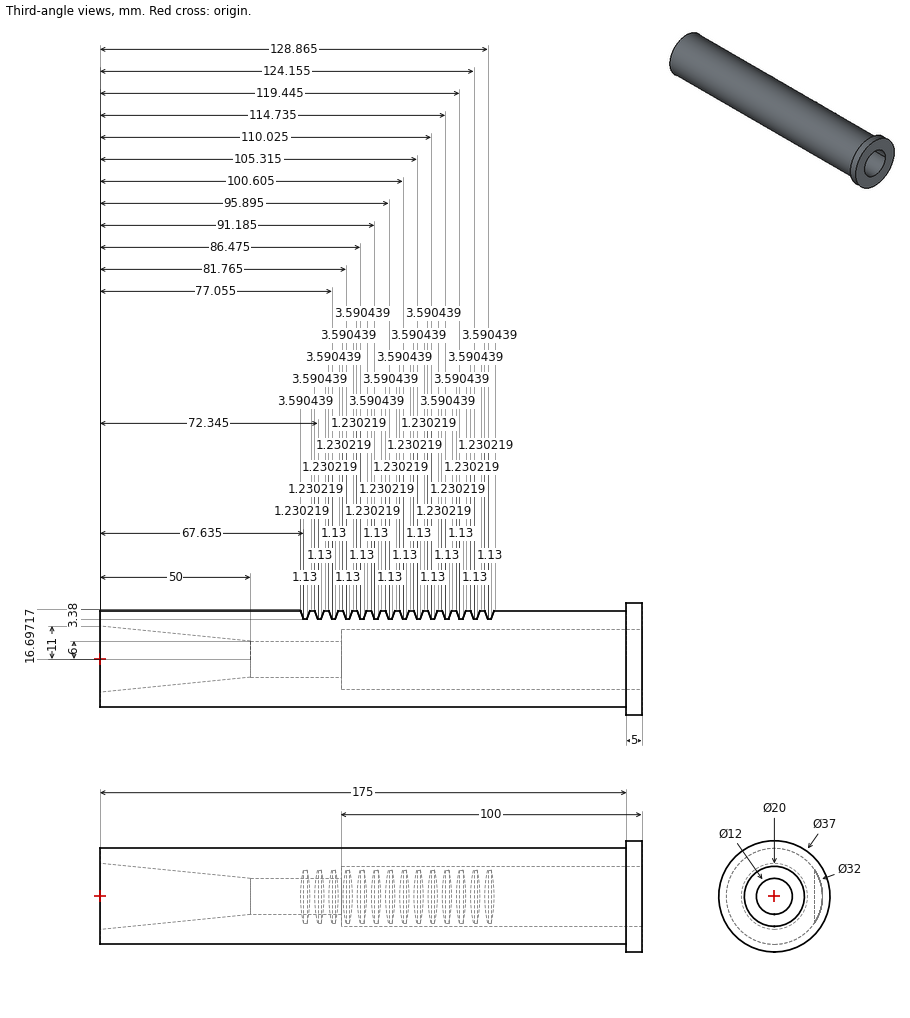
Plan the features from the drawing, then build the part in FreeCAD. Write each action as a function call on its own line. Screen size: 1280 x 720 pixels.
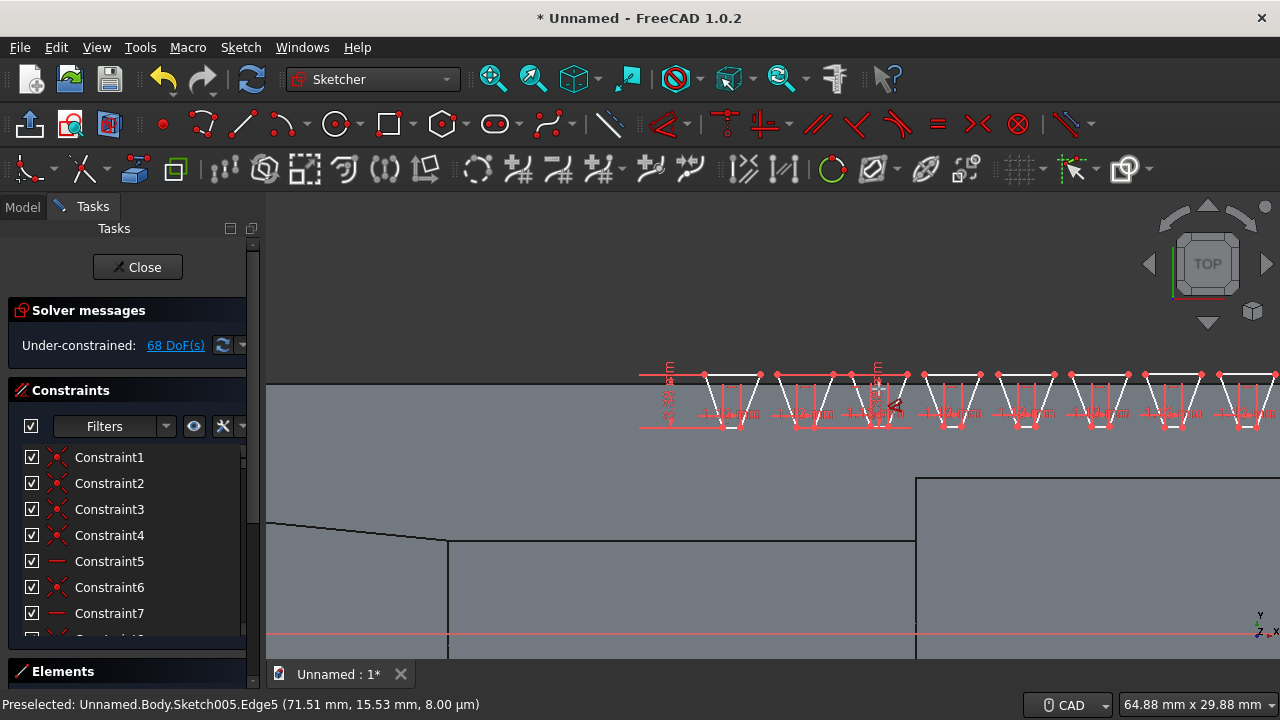
click(857, 391)
click(953, 389)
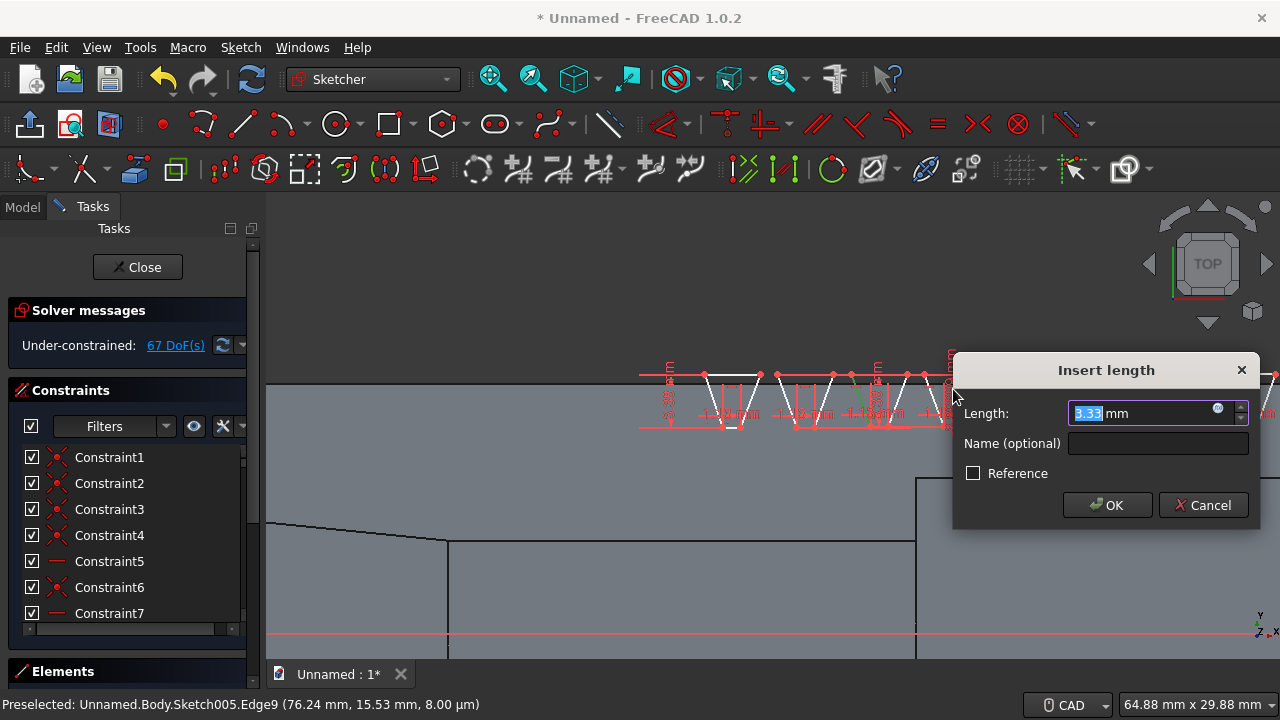
text(3.38)
key(Return)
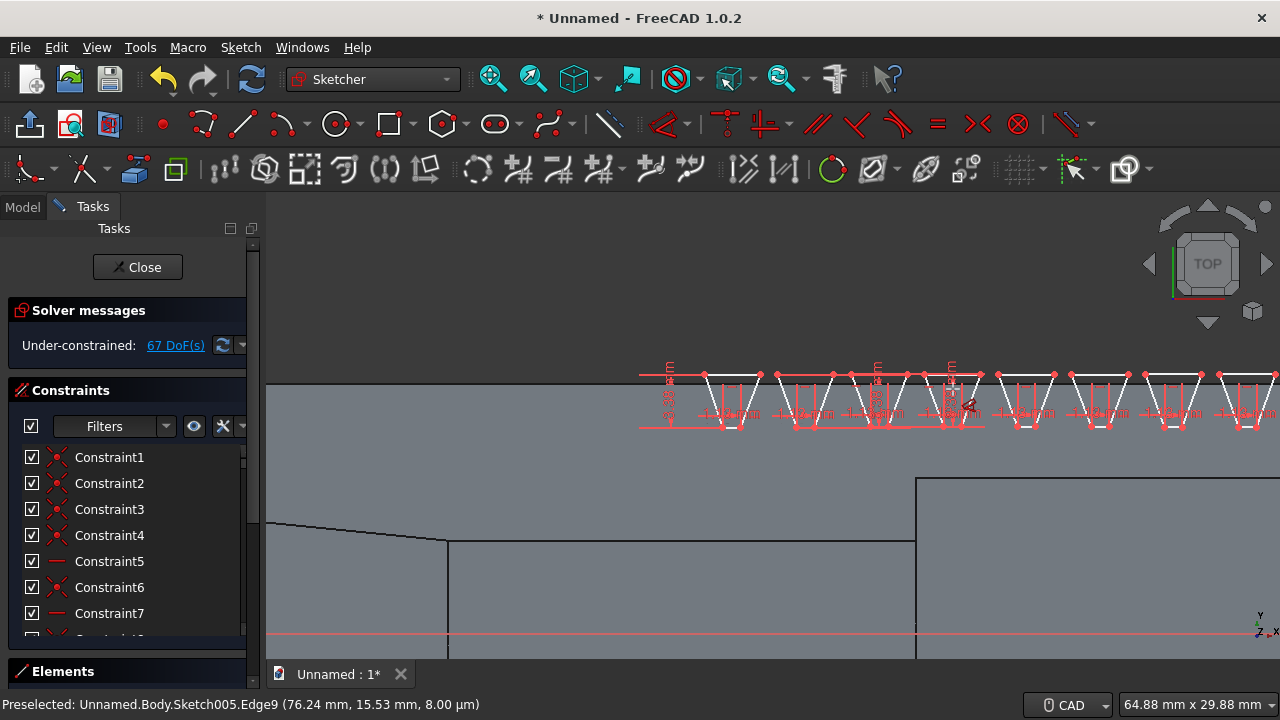
click(930, 391)
click(1026, 389)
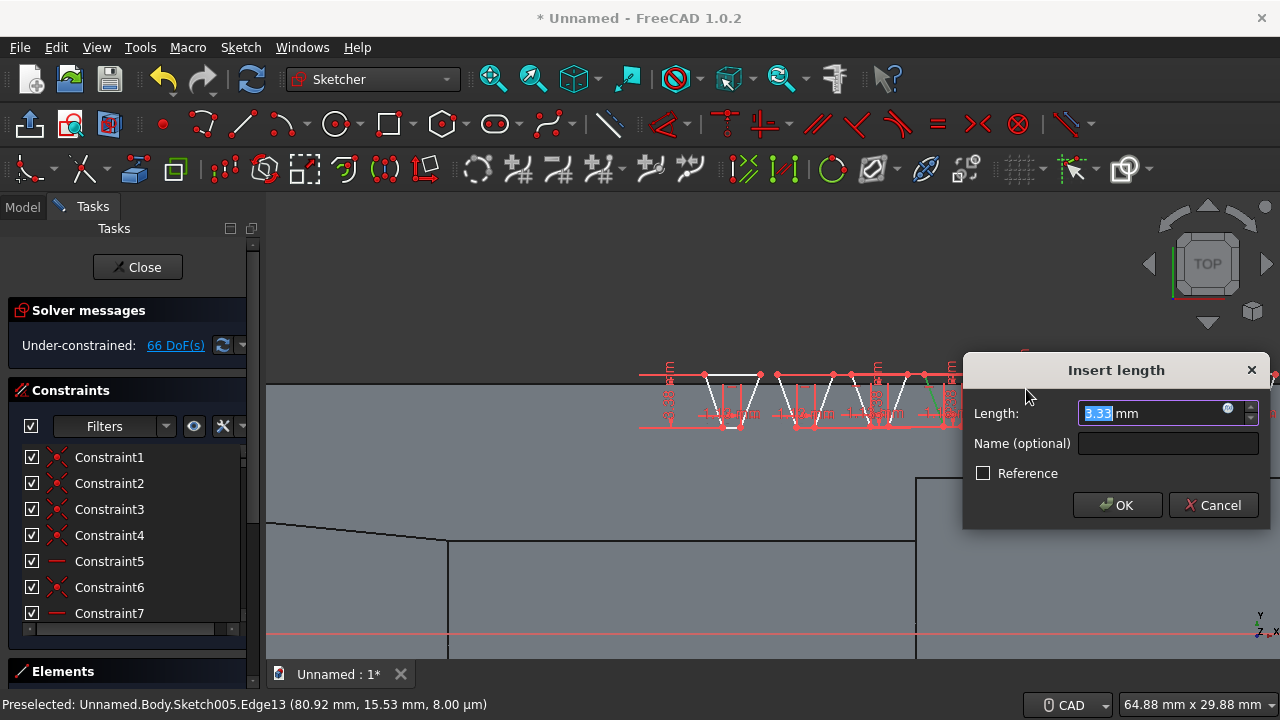
text(3.38)
key(Return)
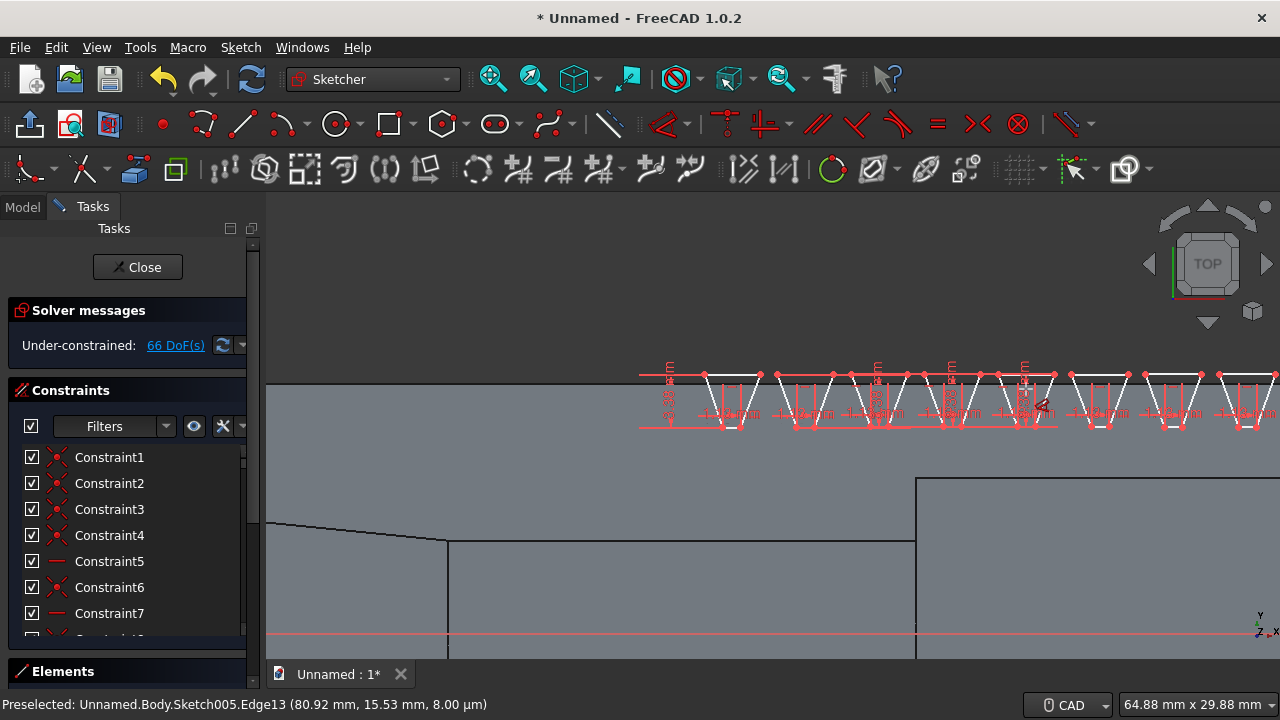
click(1004, 391)
click(1100, 389)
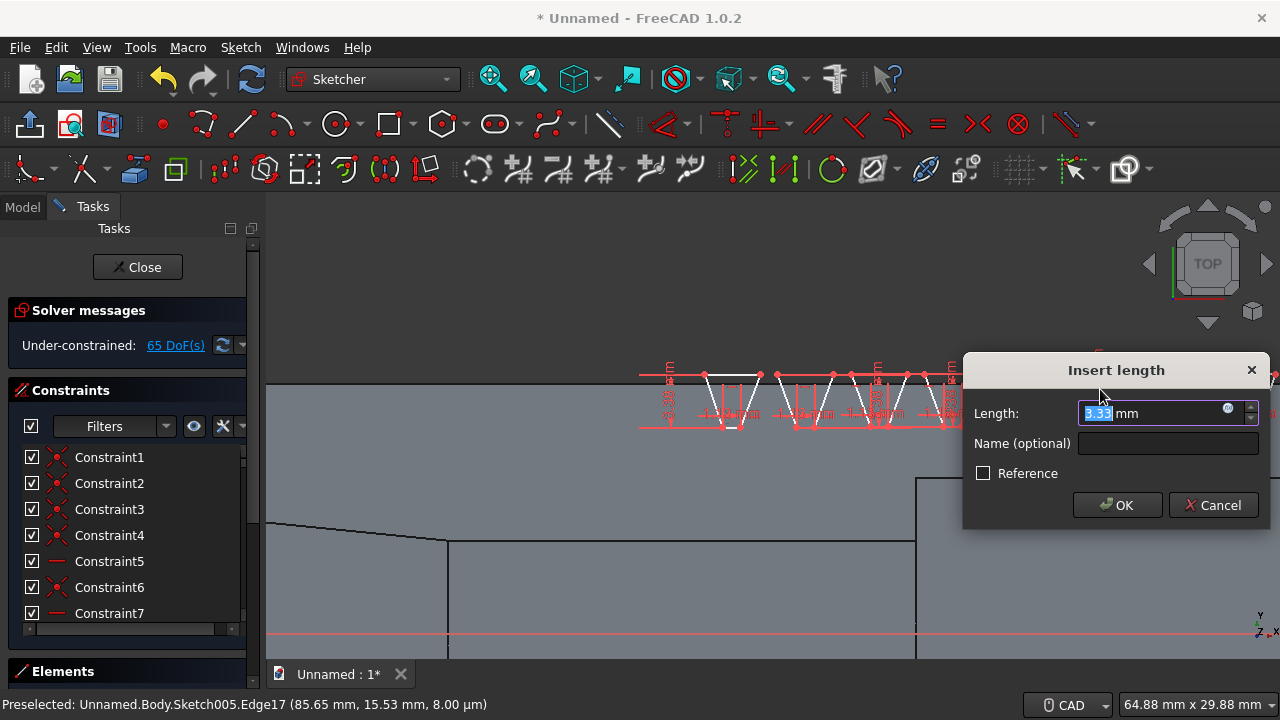
text(3.38)
key(Return)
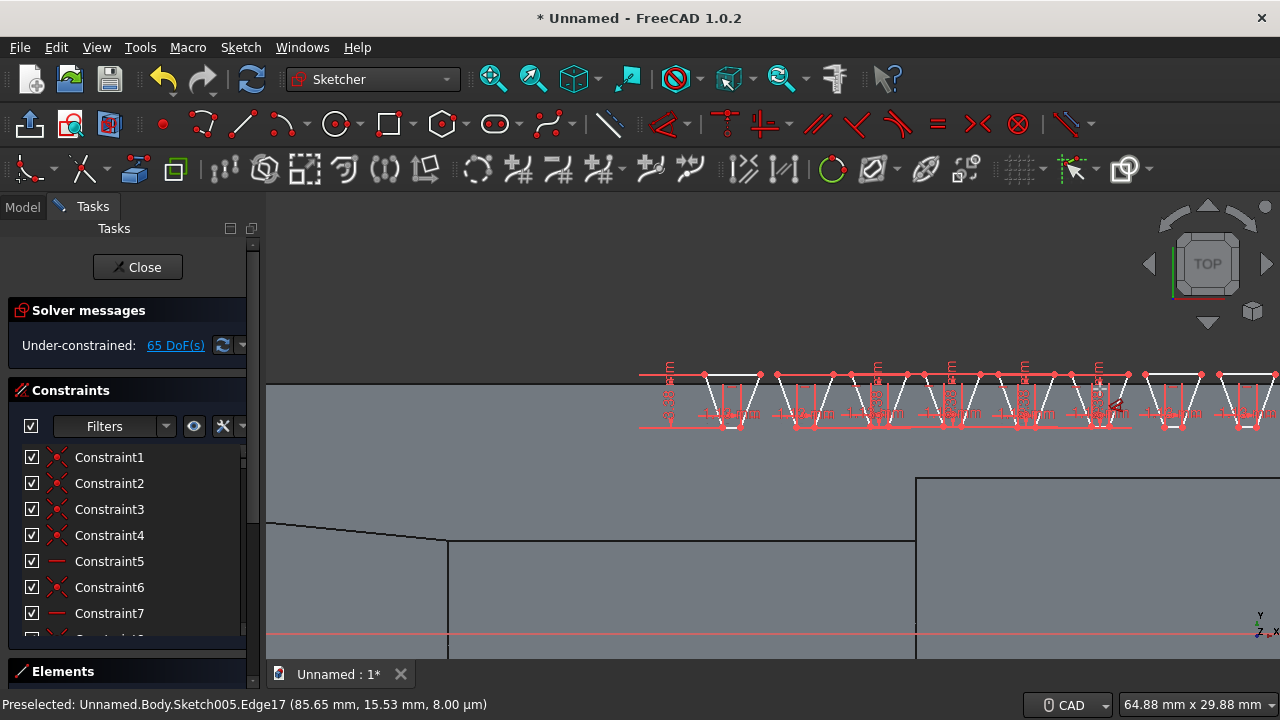
click(1078, 391)
click(1038, 401)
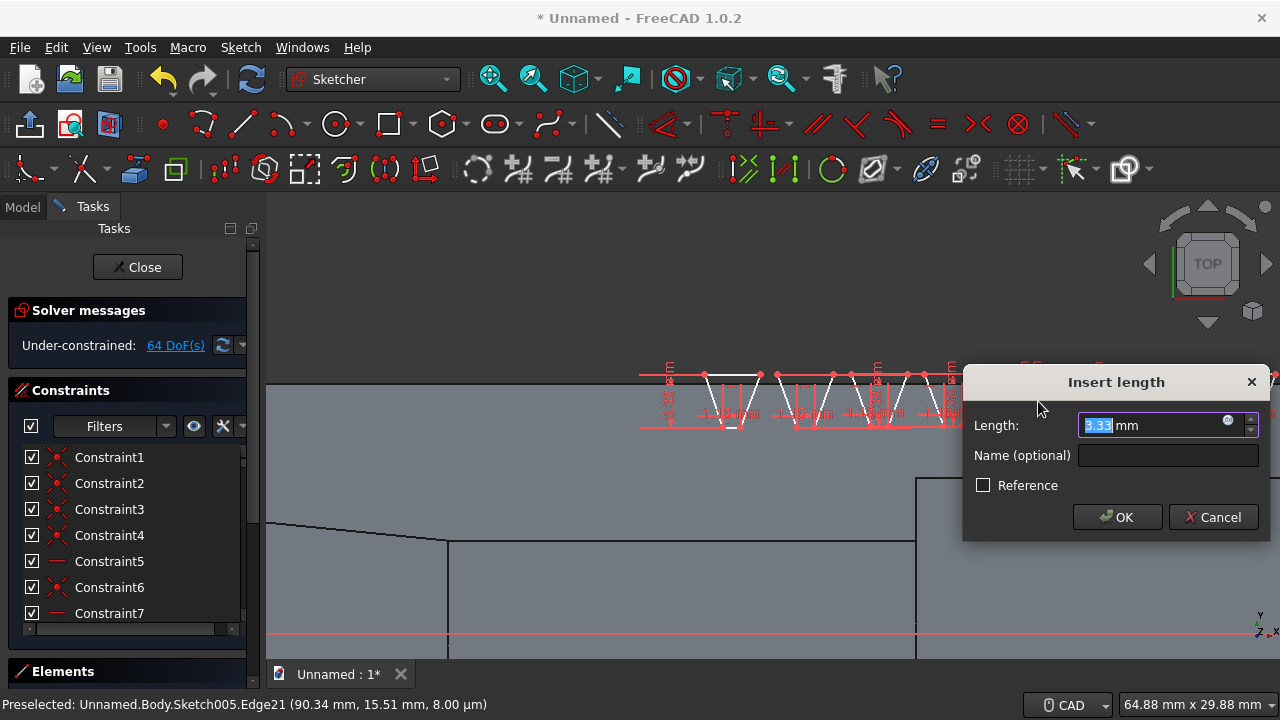
text(3.38)
key(Return)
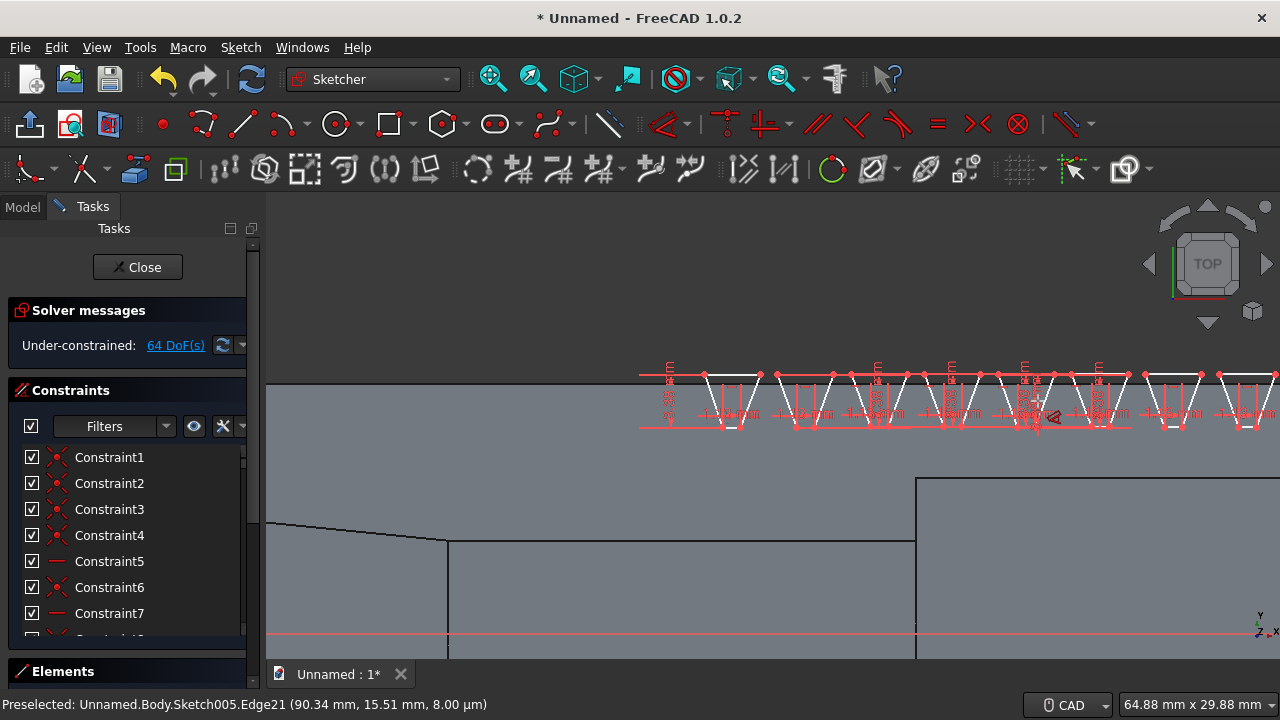
scroll(710, 392, down, 6)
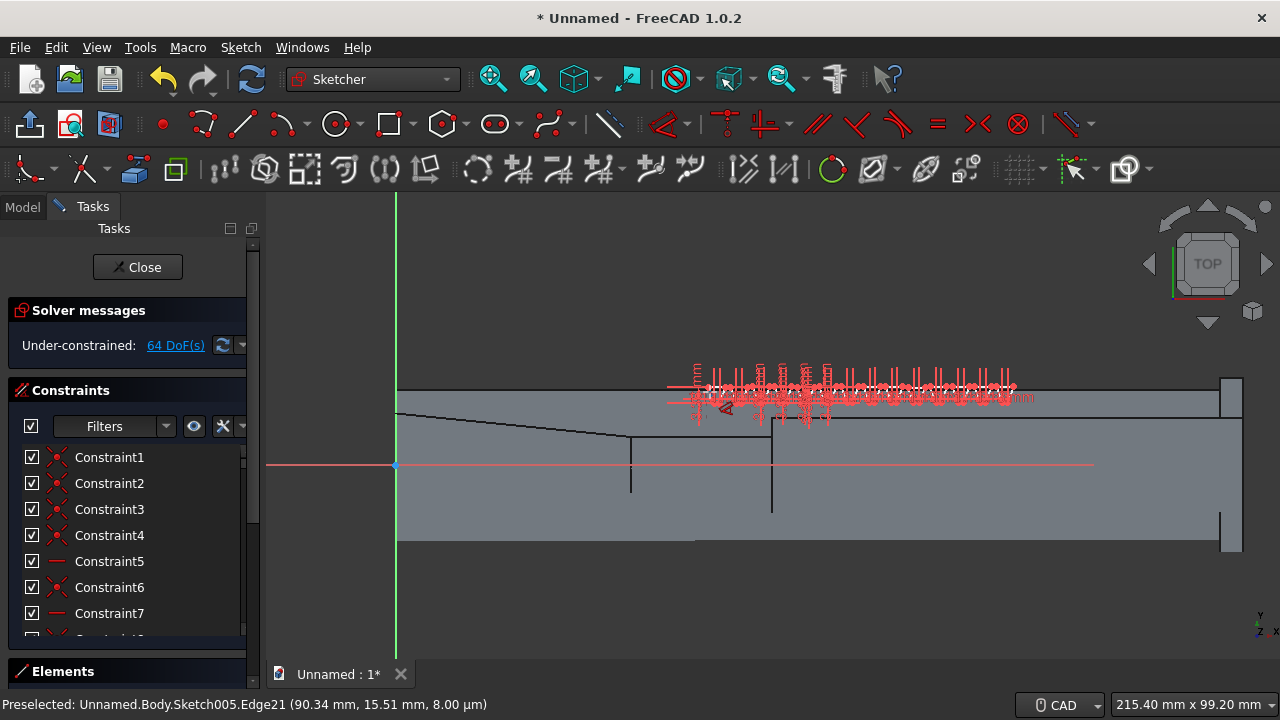
scroll(843, 392, up, 6)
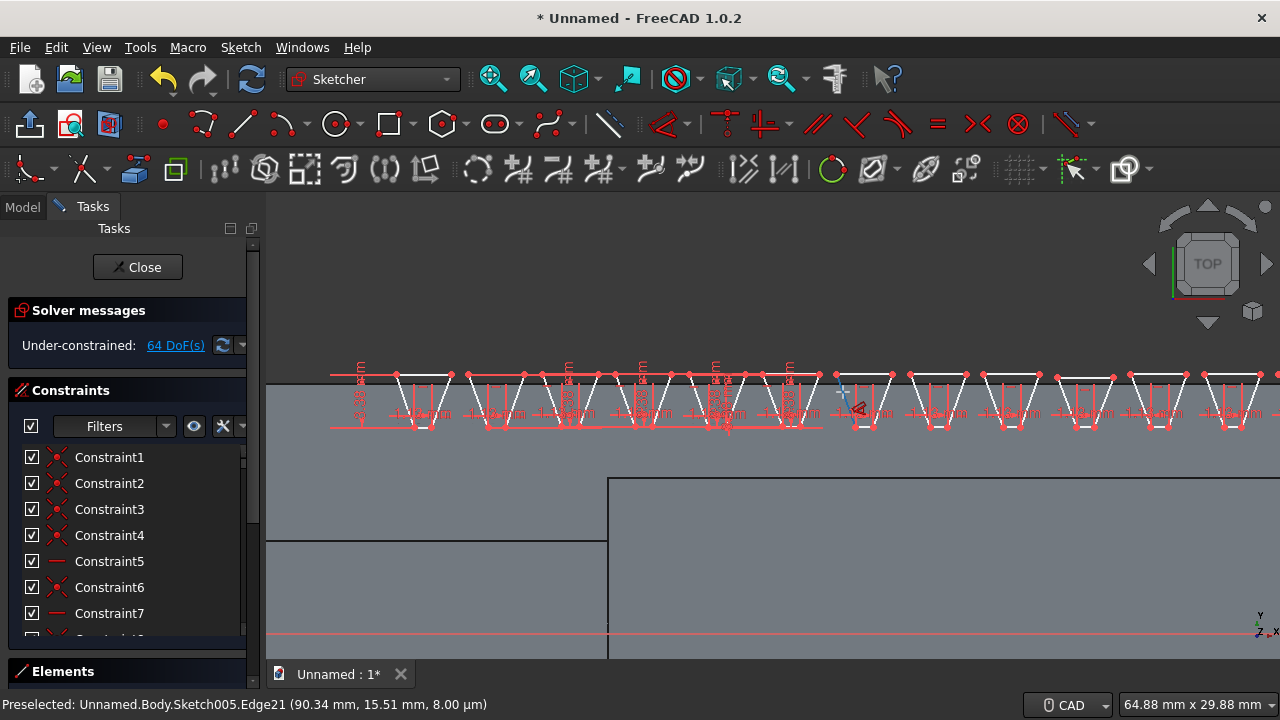
click(842, 390)
click(938, 389)